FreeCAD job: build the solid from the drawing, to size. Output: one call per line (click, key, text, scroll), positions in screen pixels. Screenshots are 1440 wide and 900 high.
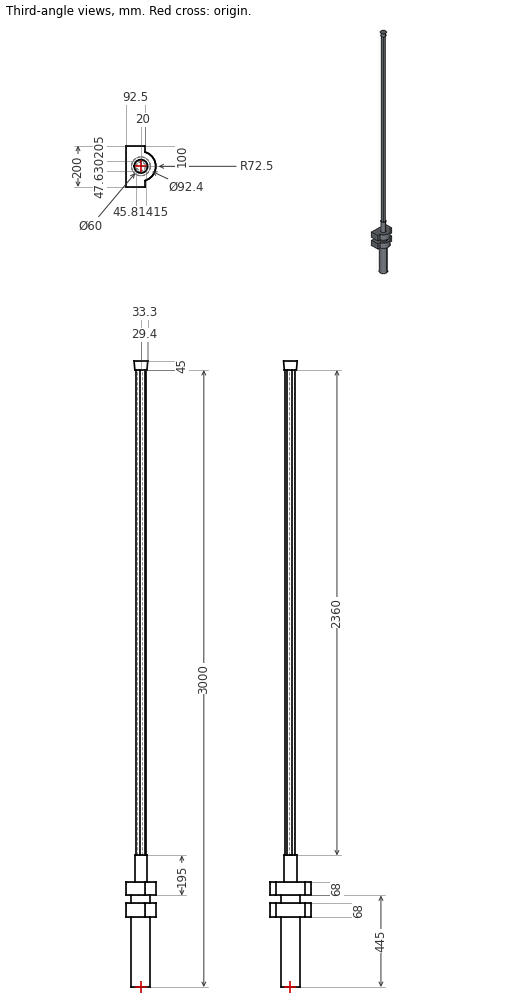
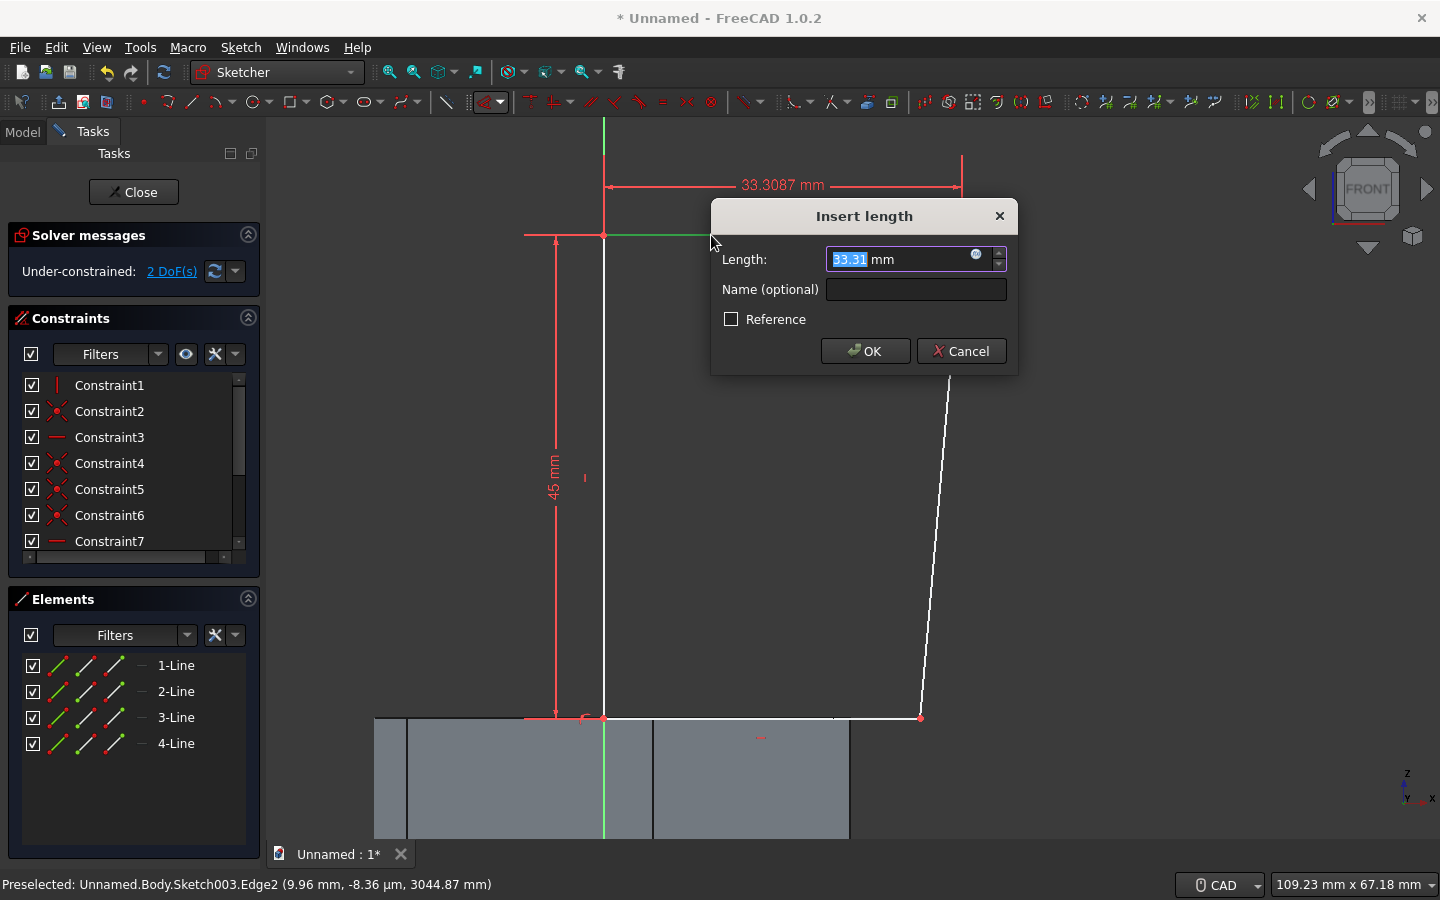
text(33.3)
key(Return)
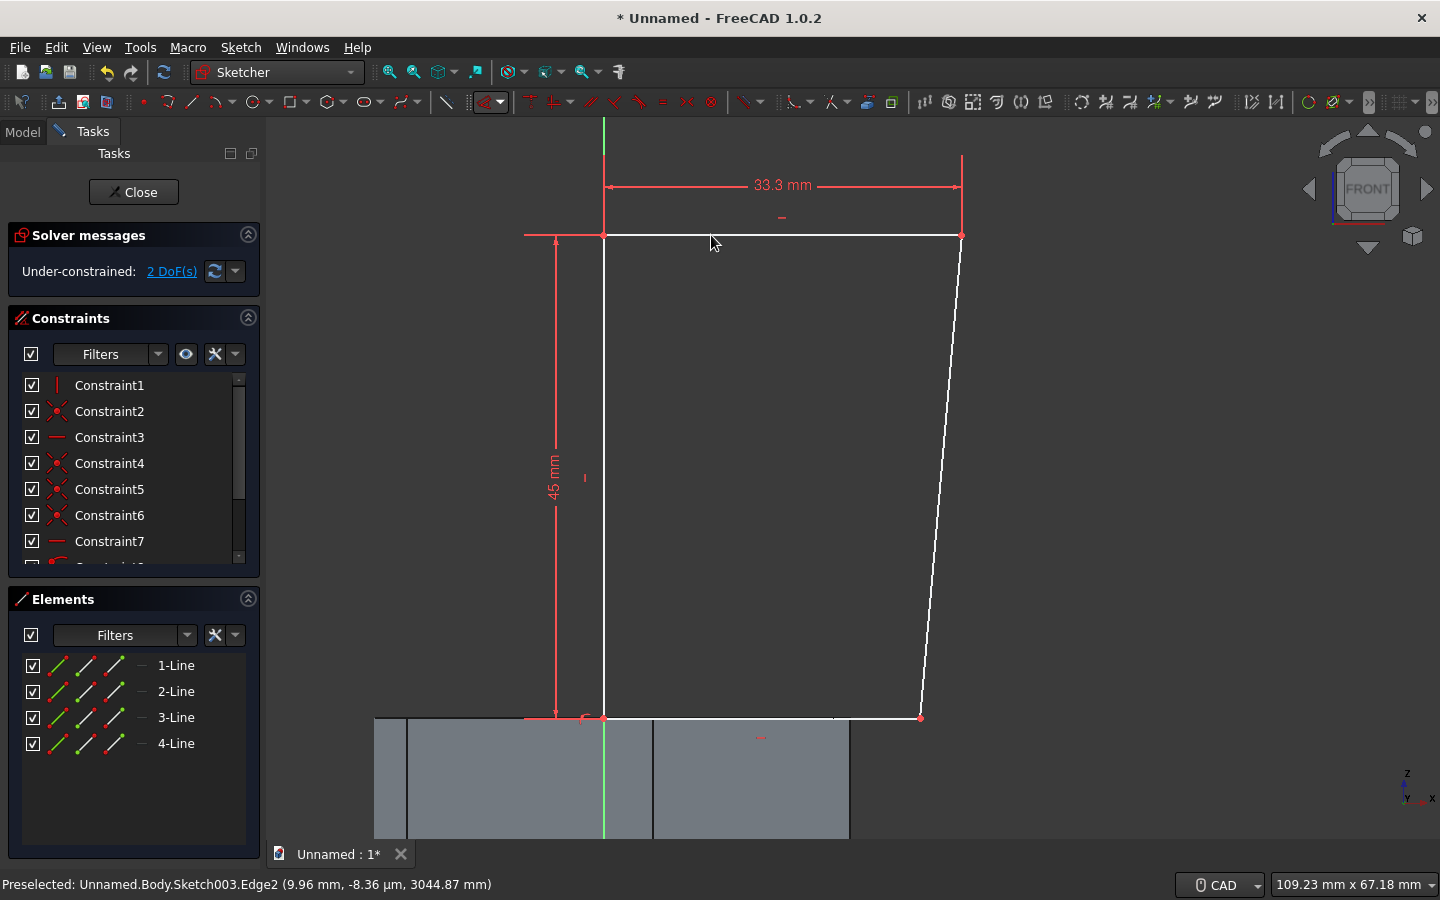
click(825, 719)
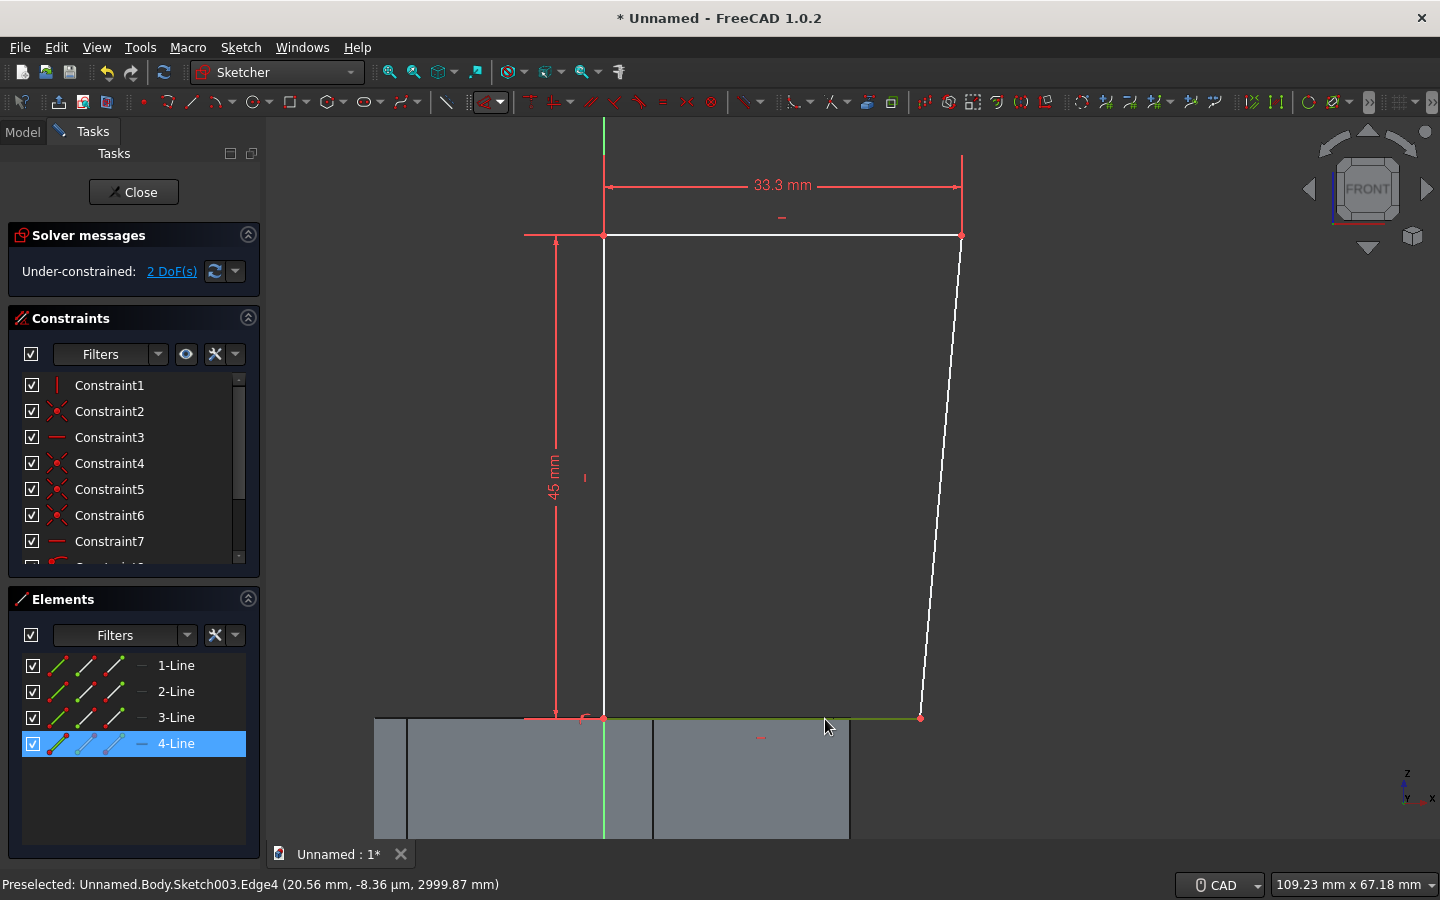
key(l)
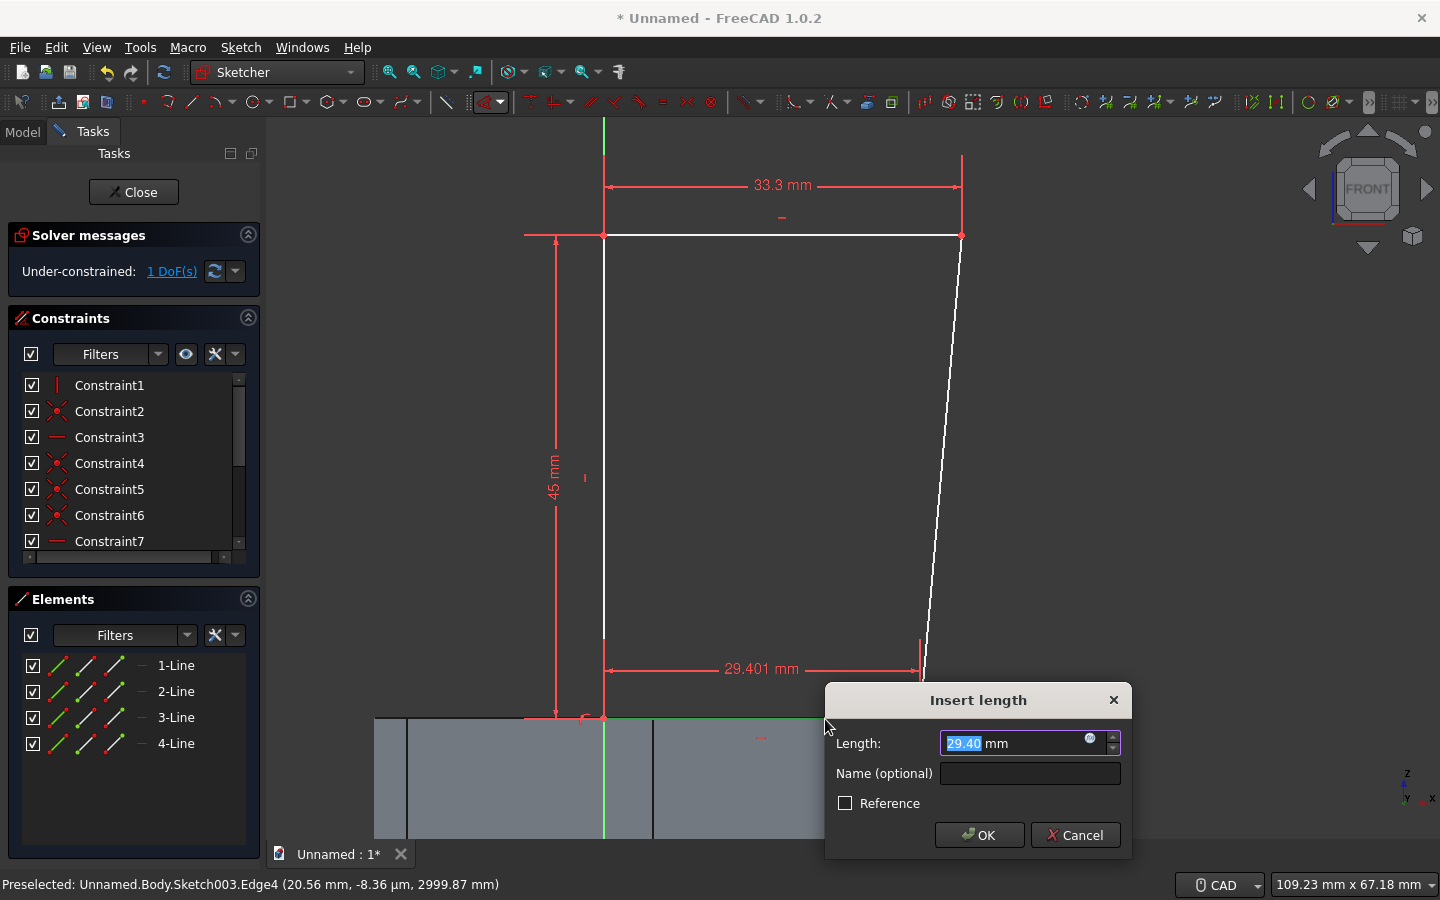
text(29.4)
key(Return)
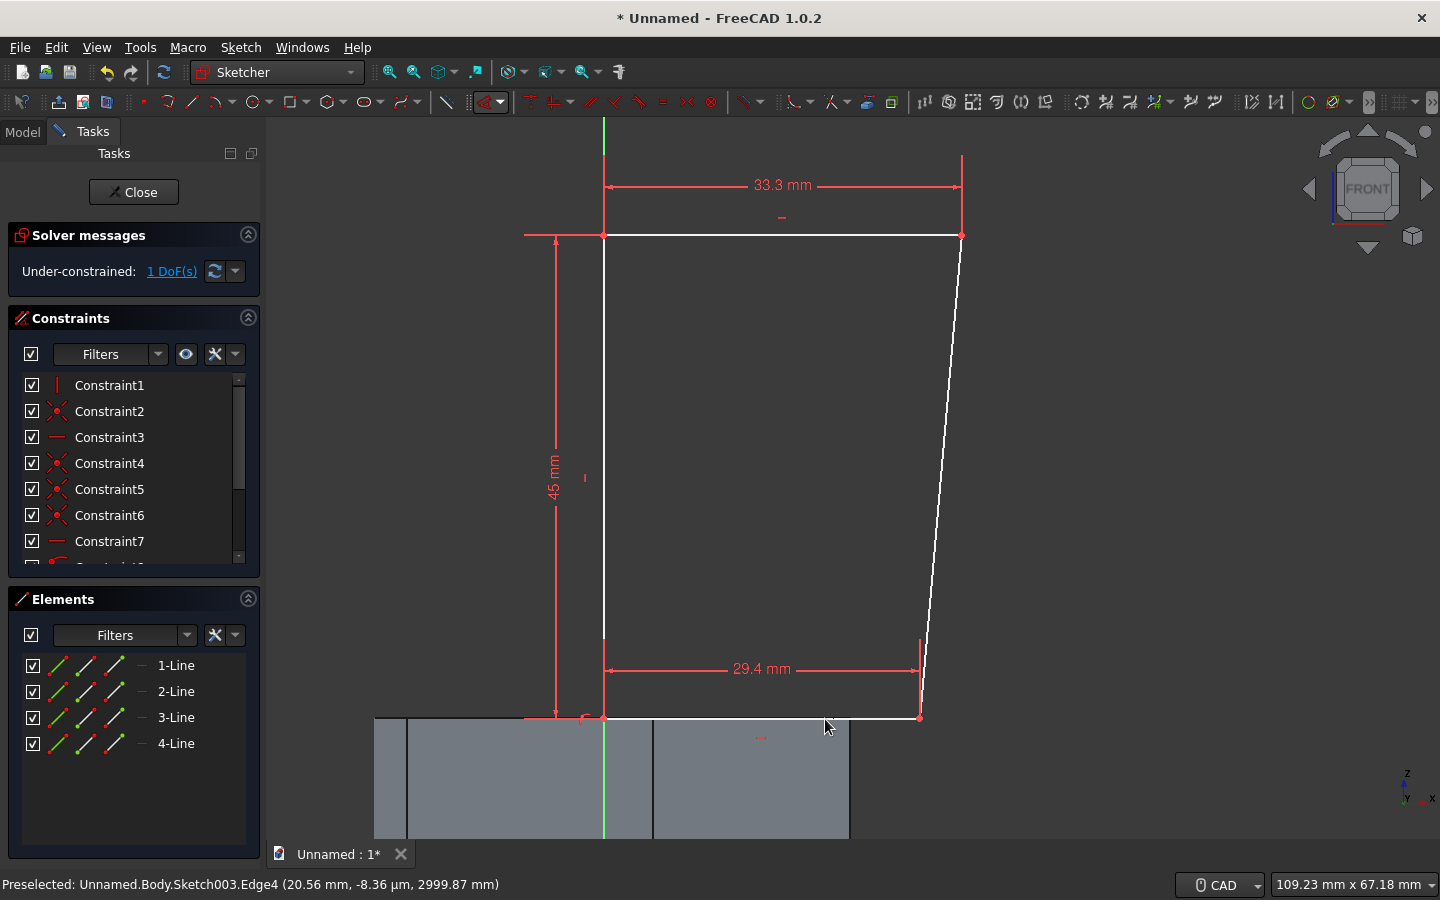
click(604, 719)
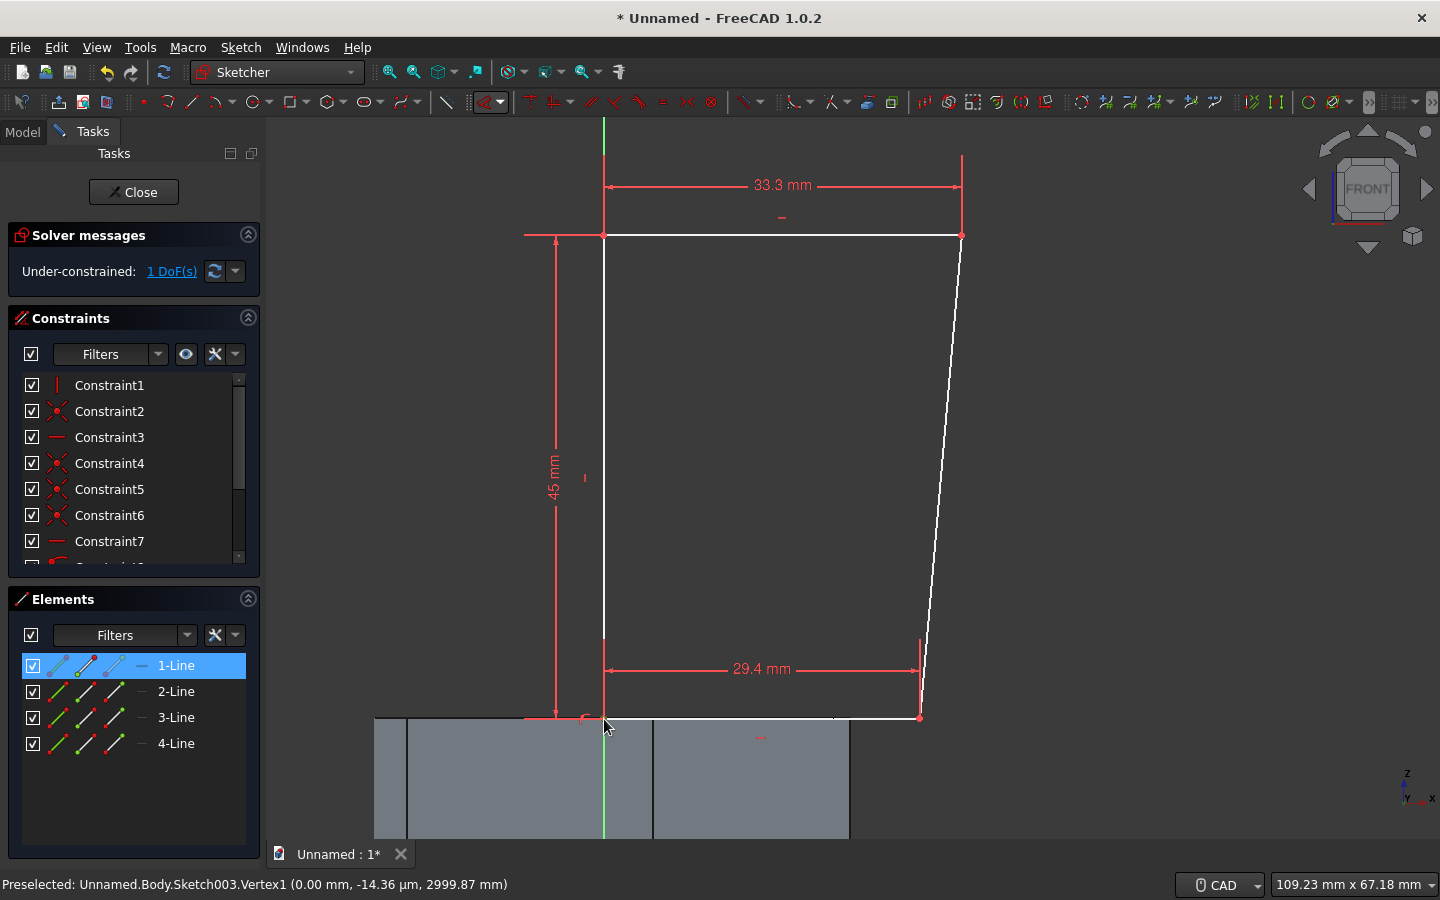
key(i)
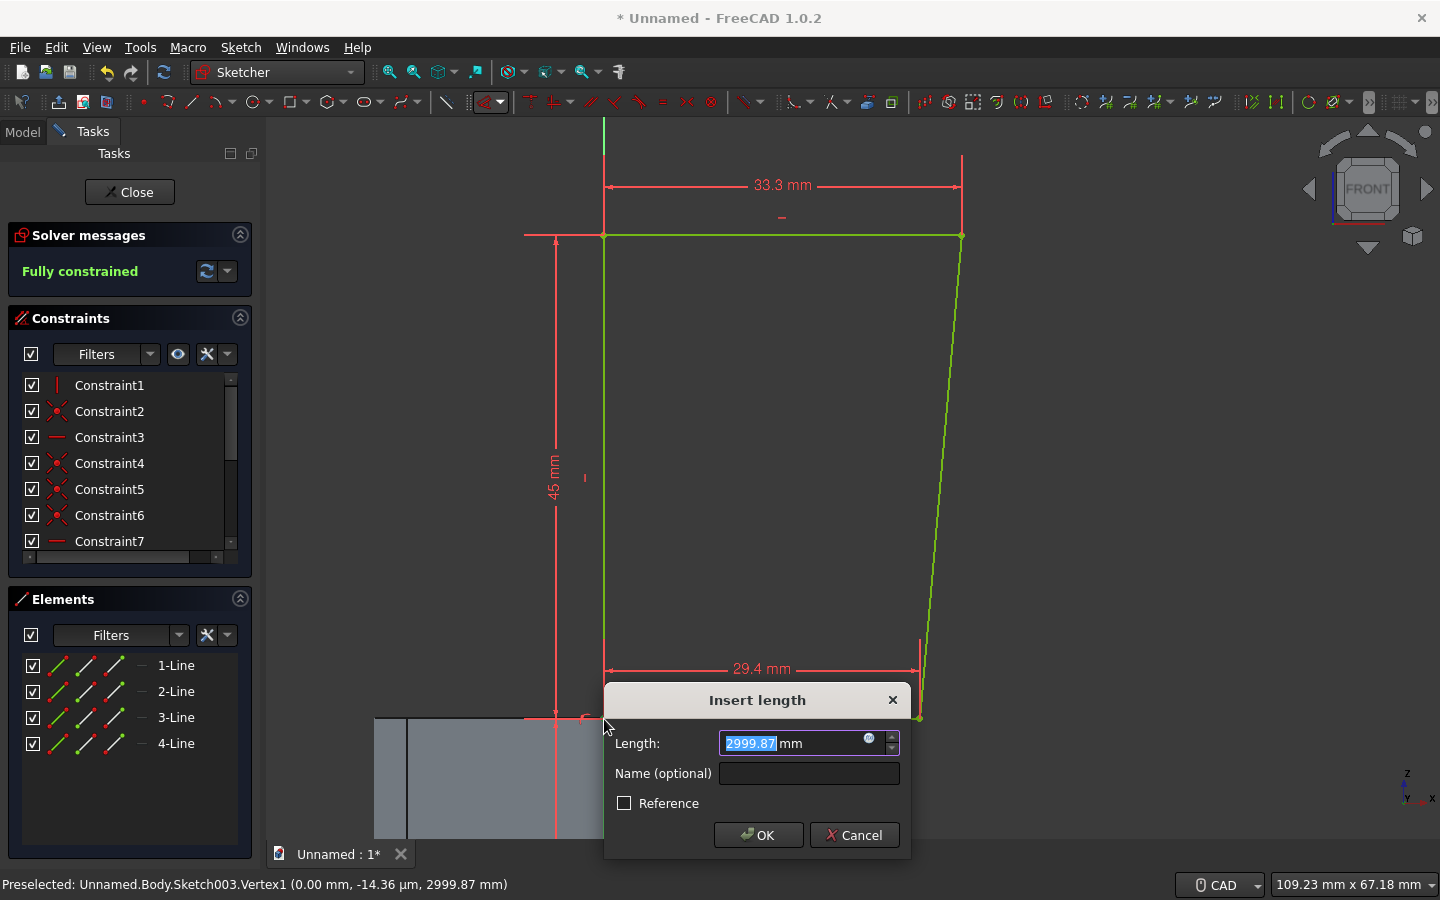
text(3000)
key(Return)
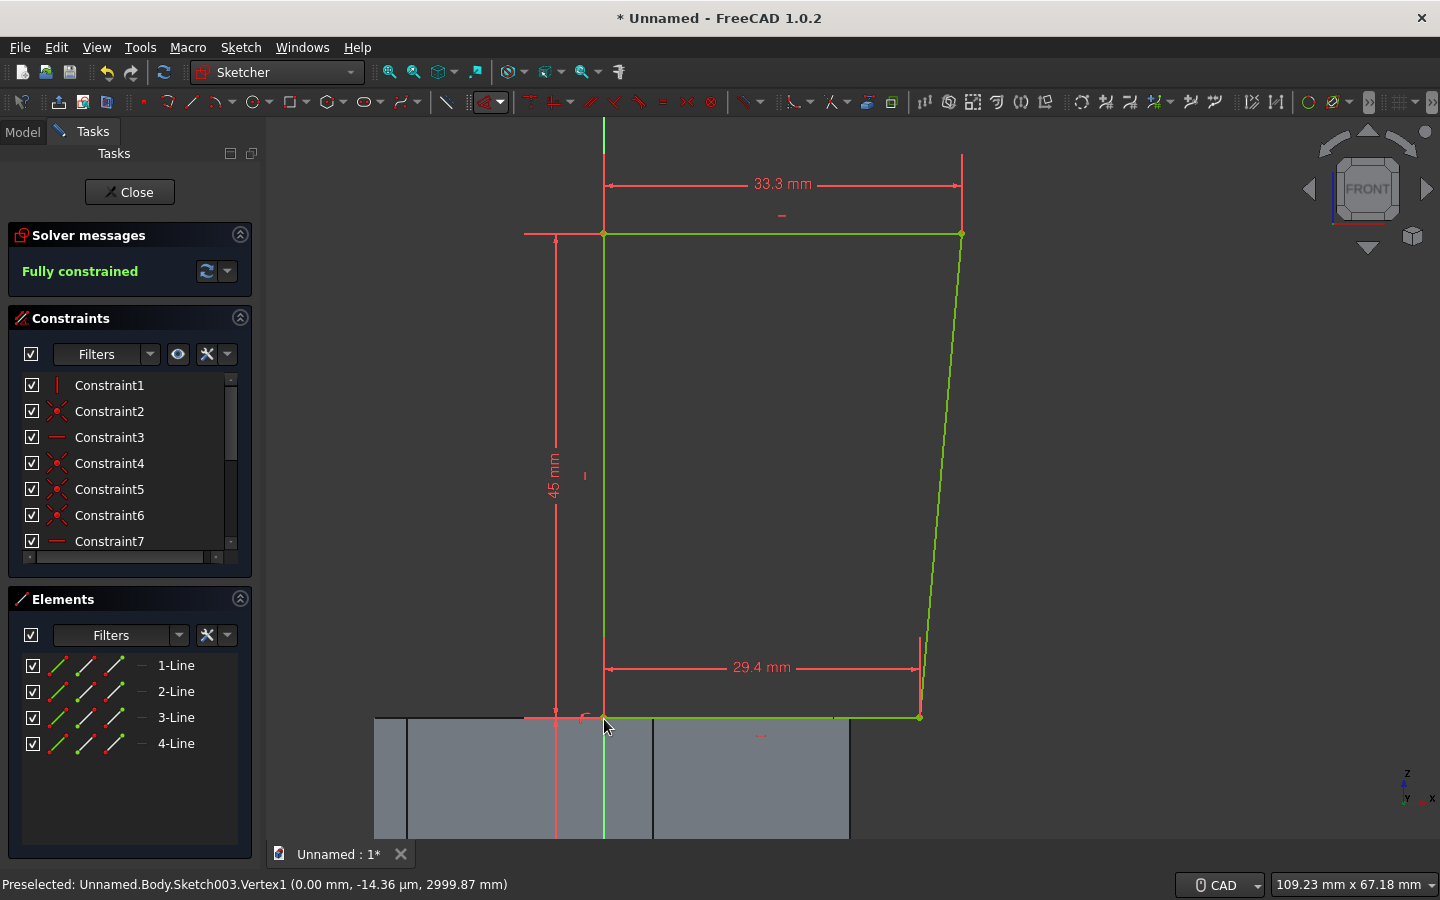
click(130, 192)